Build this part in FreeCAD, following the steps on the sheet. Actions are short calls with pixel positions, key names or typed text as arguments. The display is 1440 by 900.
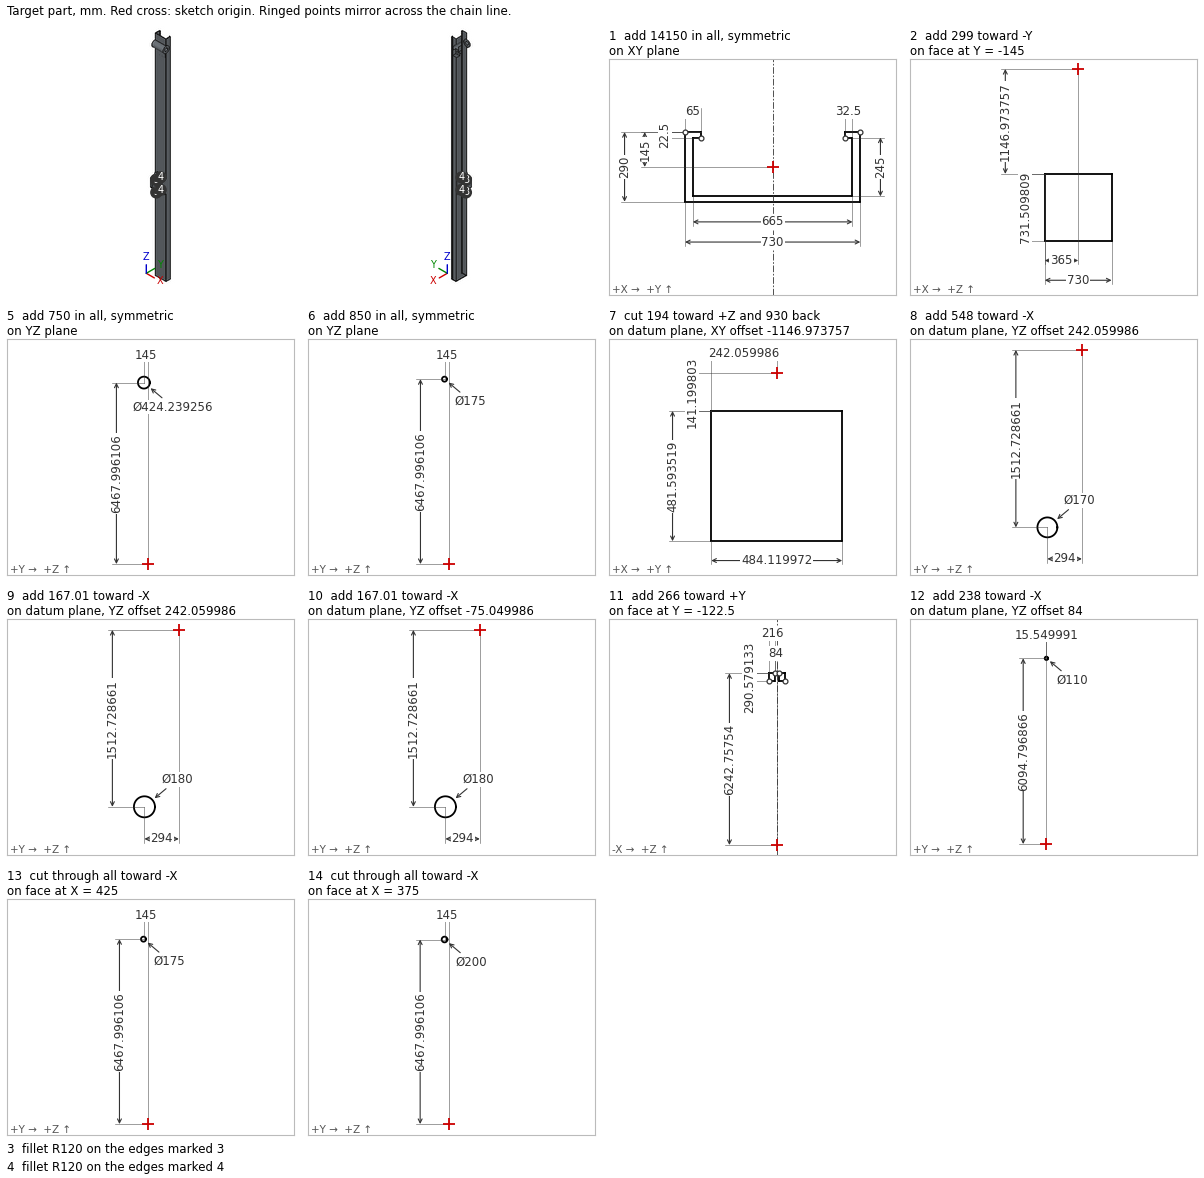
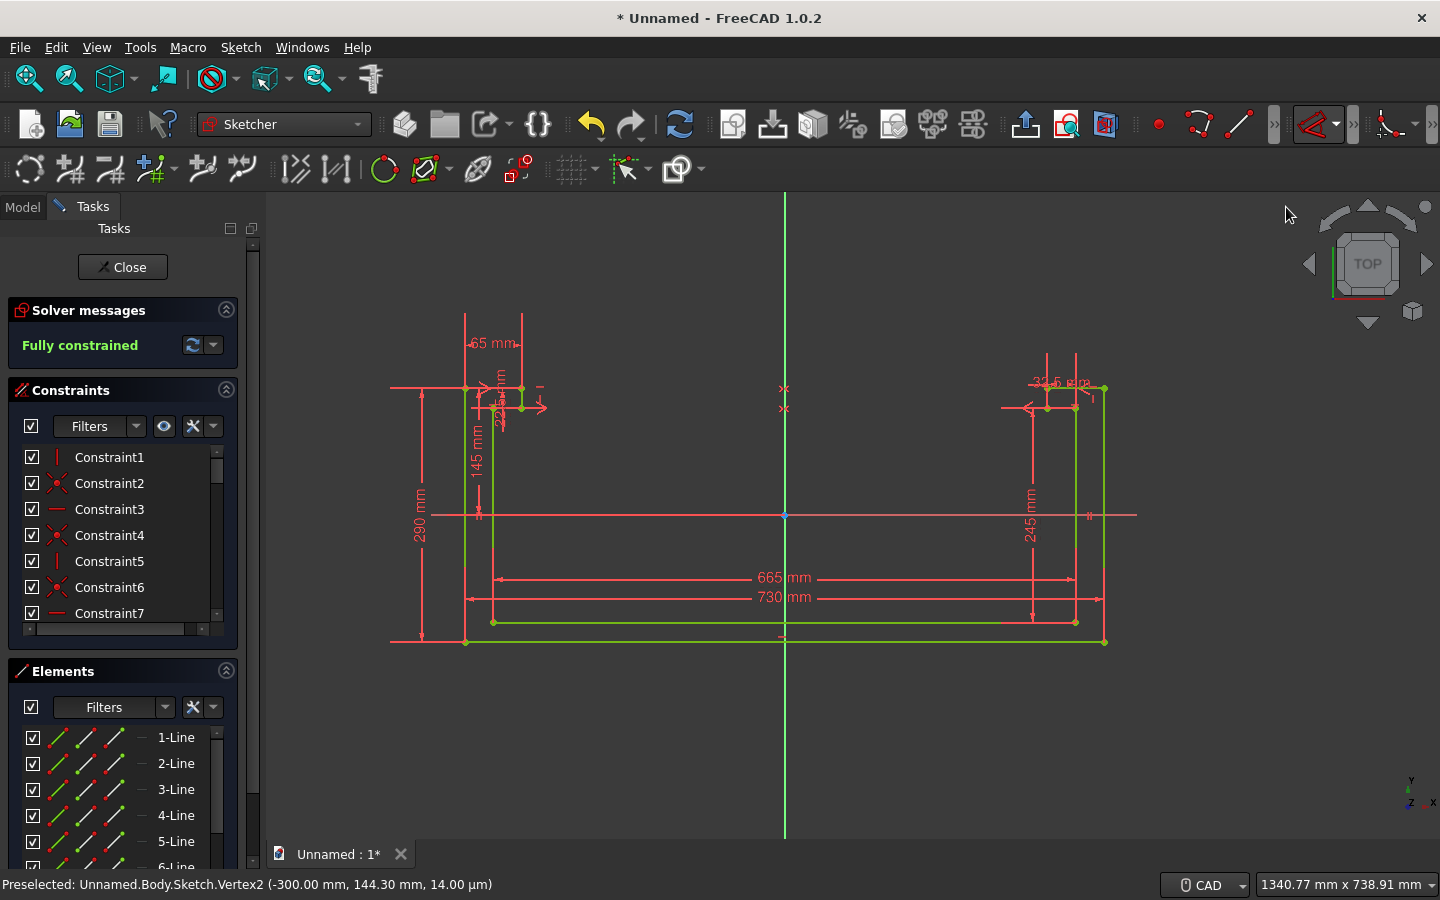
click(123, 267)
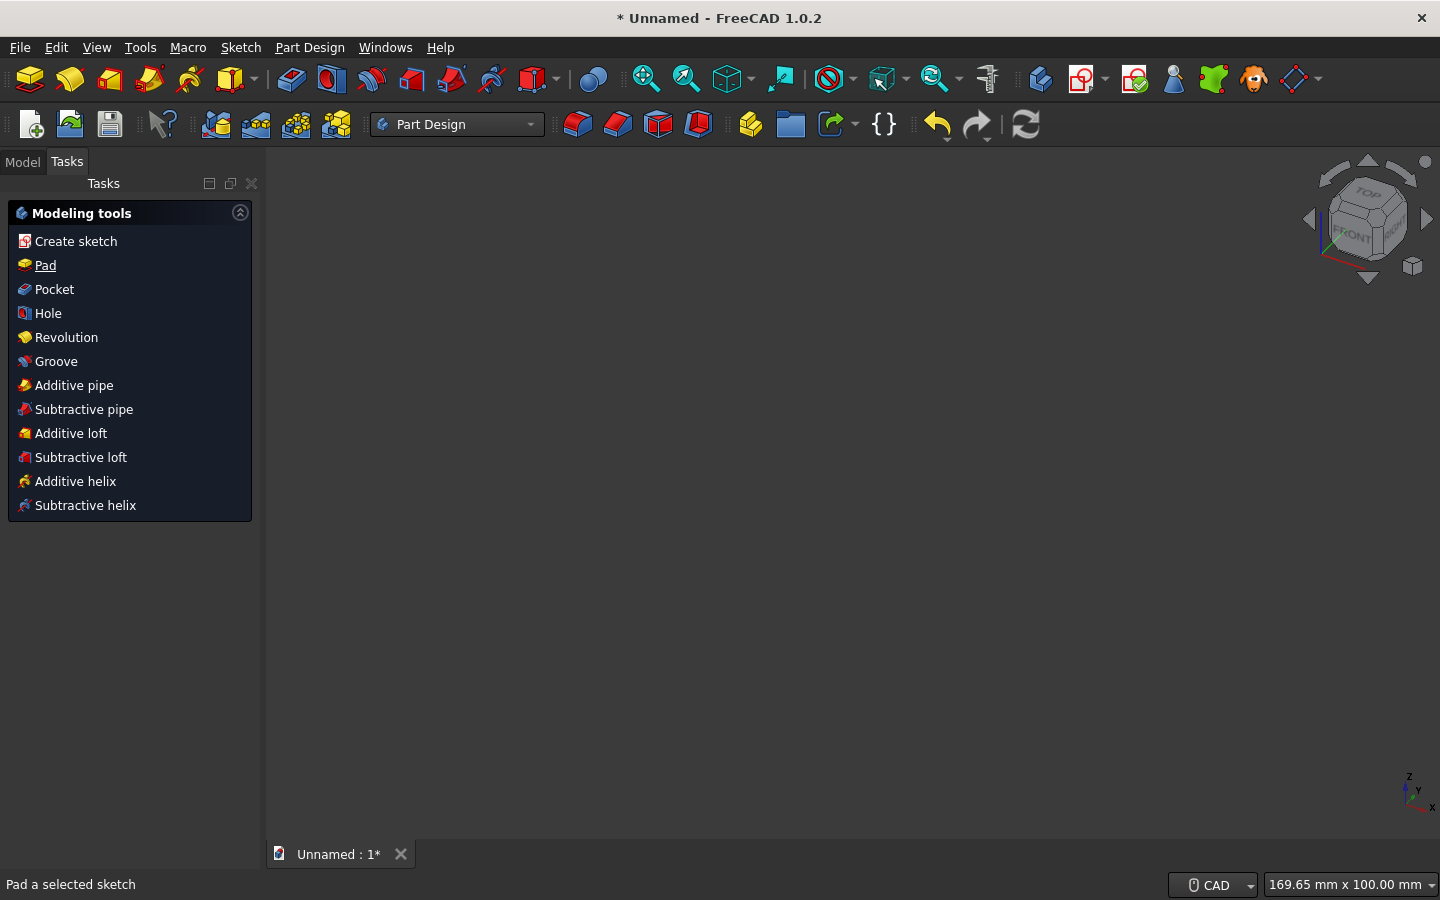
click(30, 80)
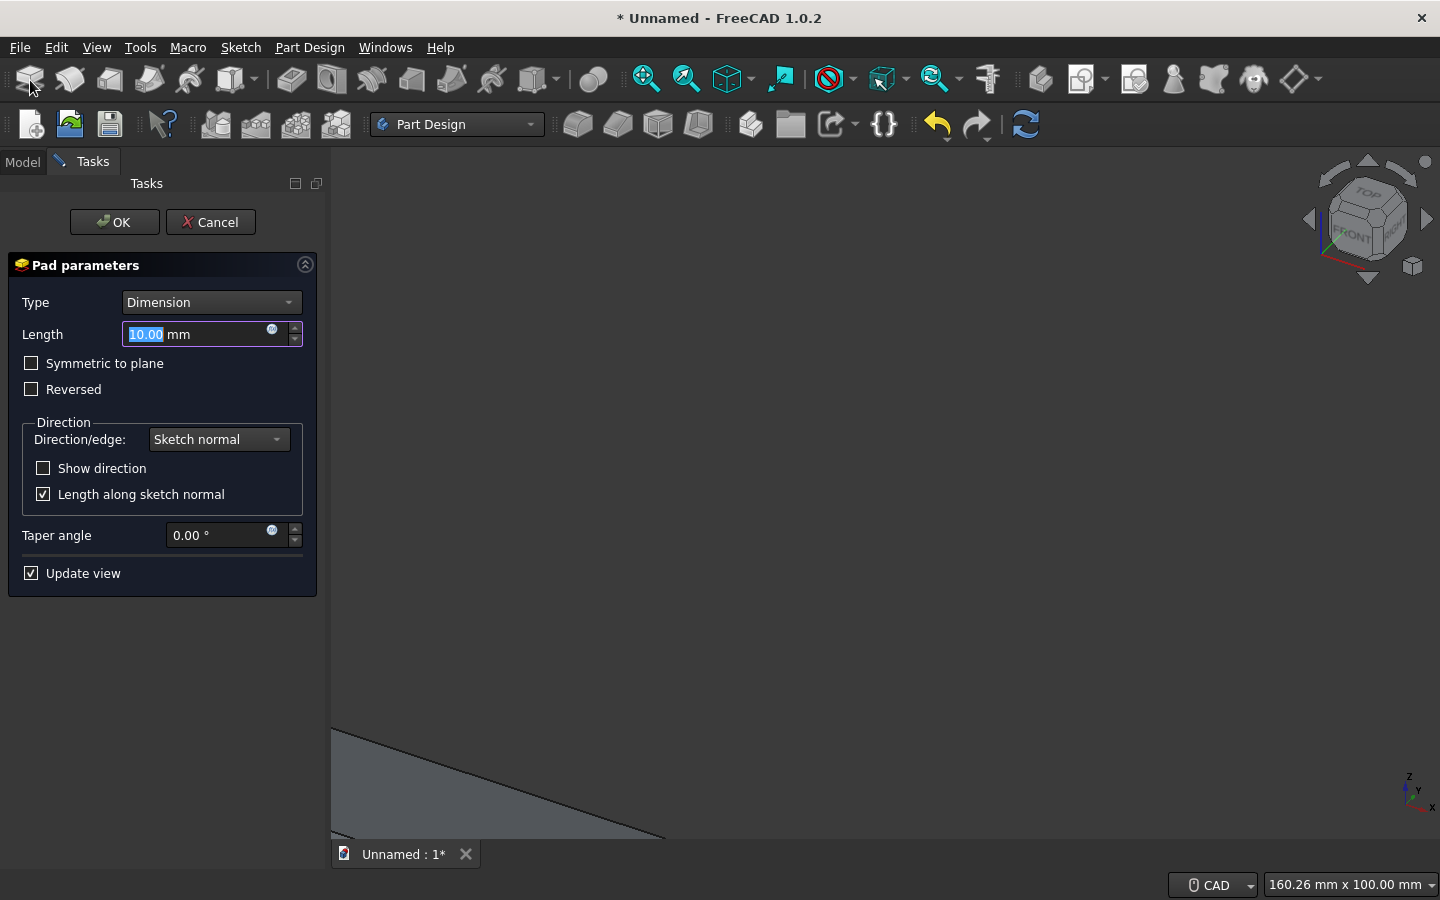
text(14150)
key(Tab)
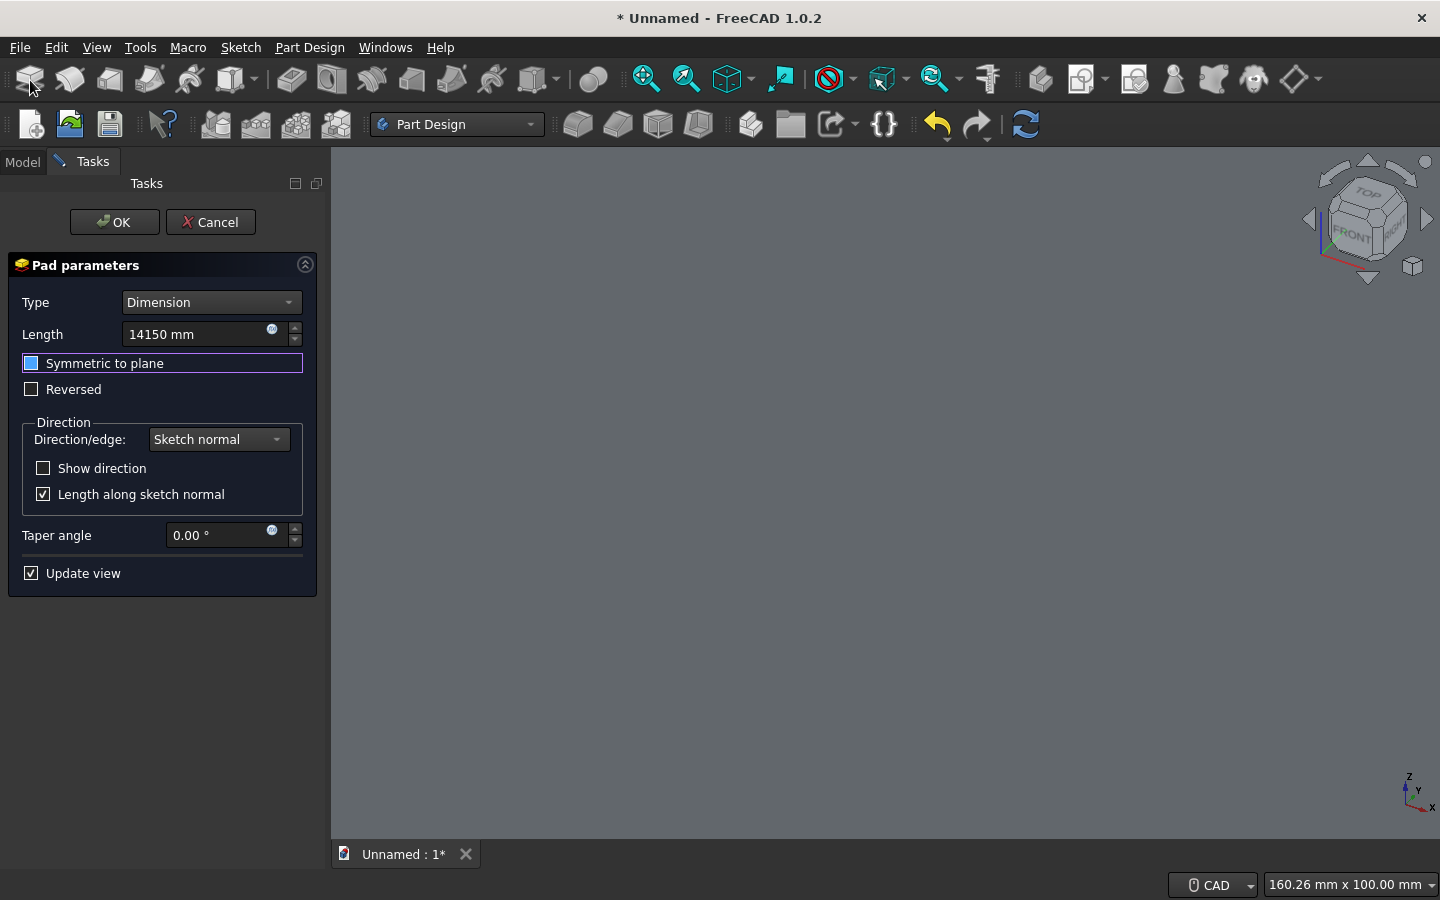
click(30, 363)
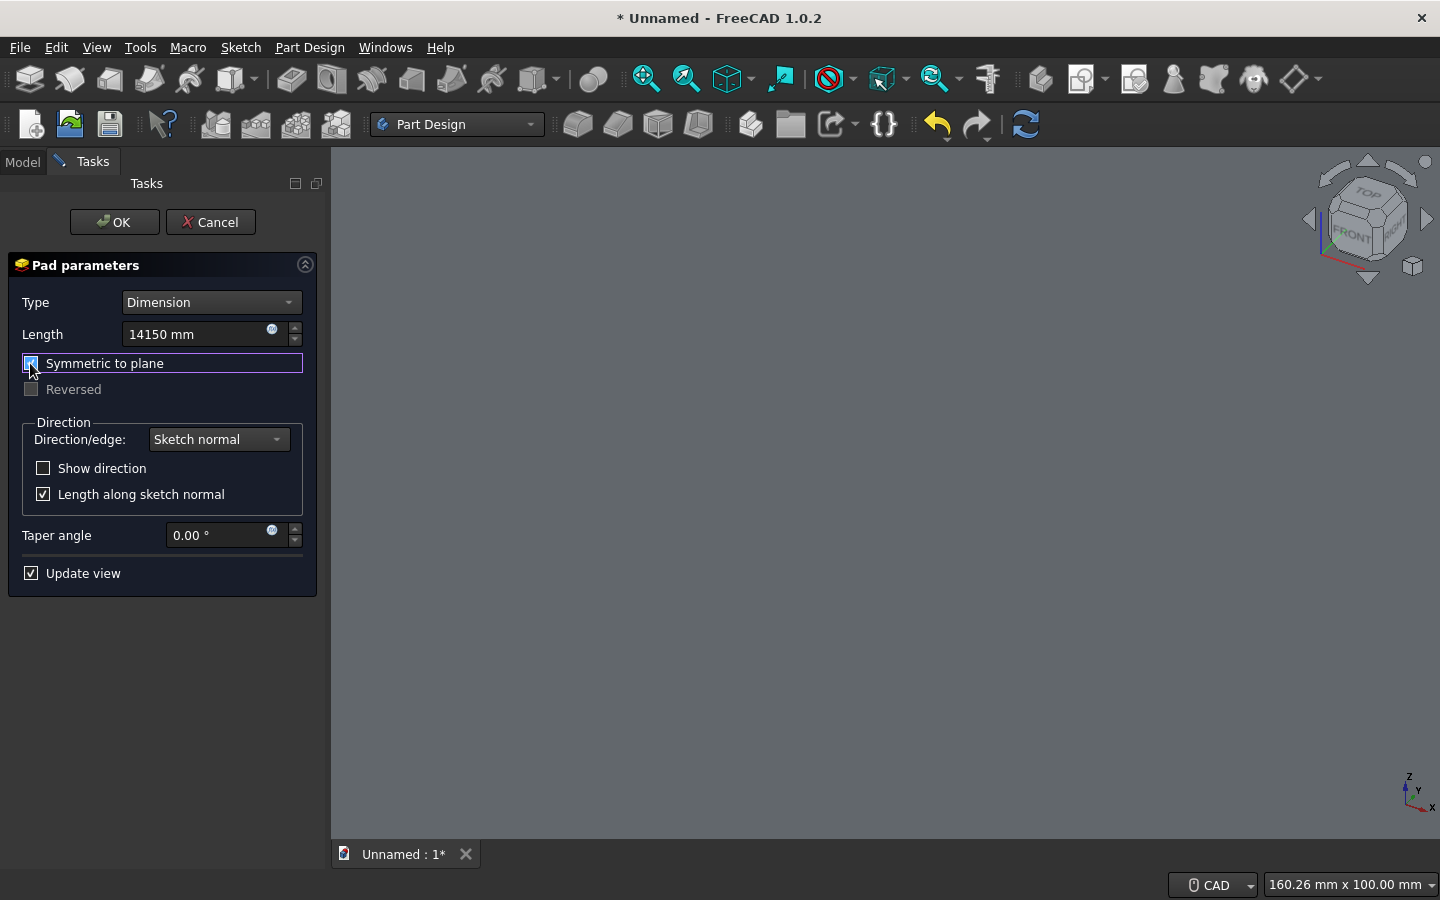
click(115, 222)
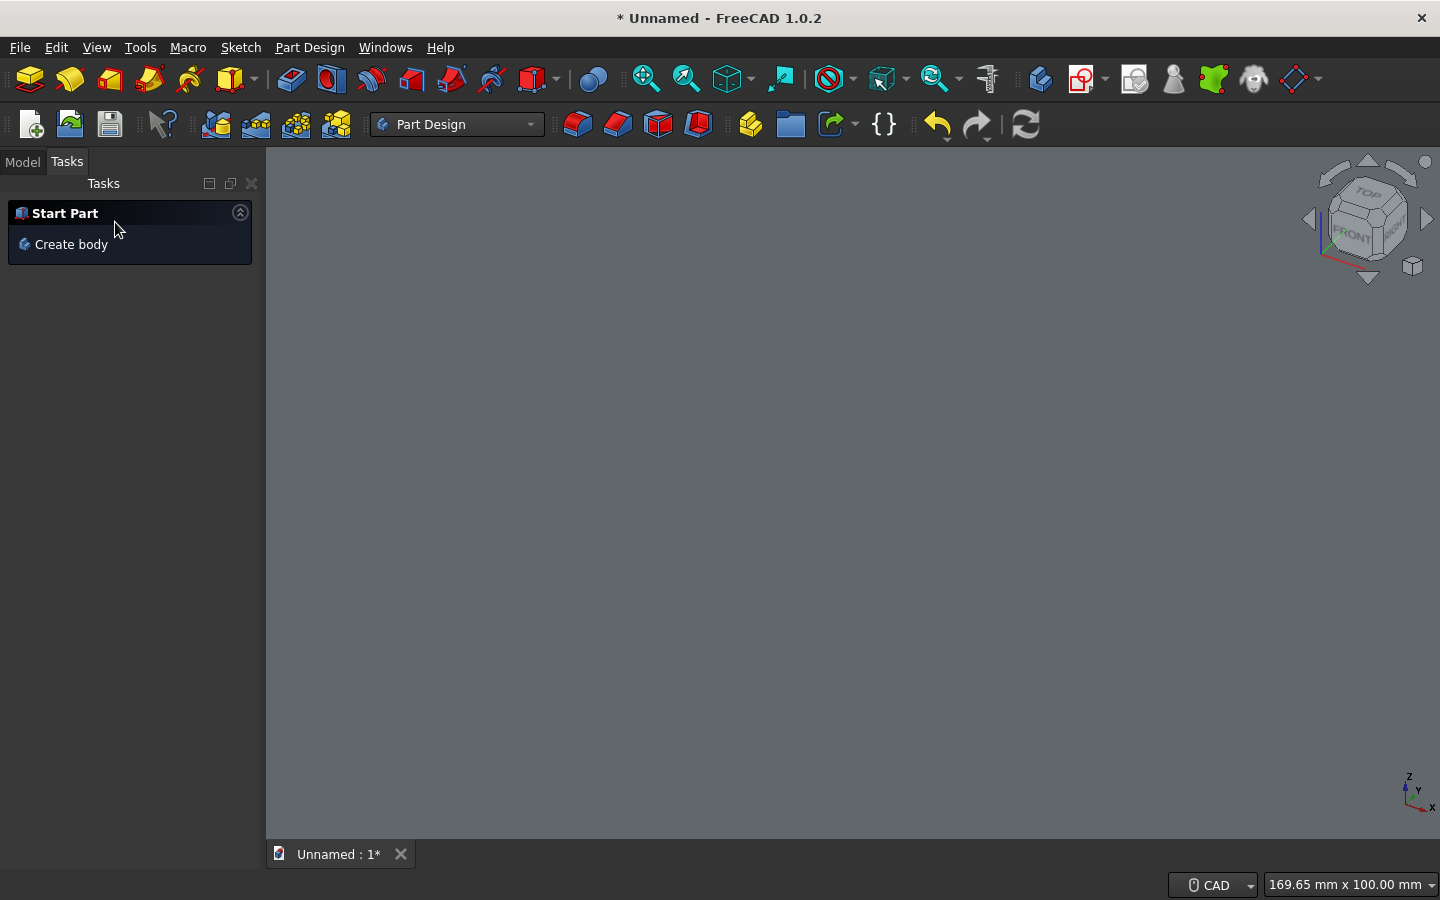
key(v)
key(f)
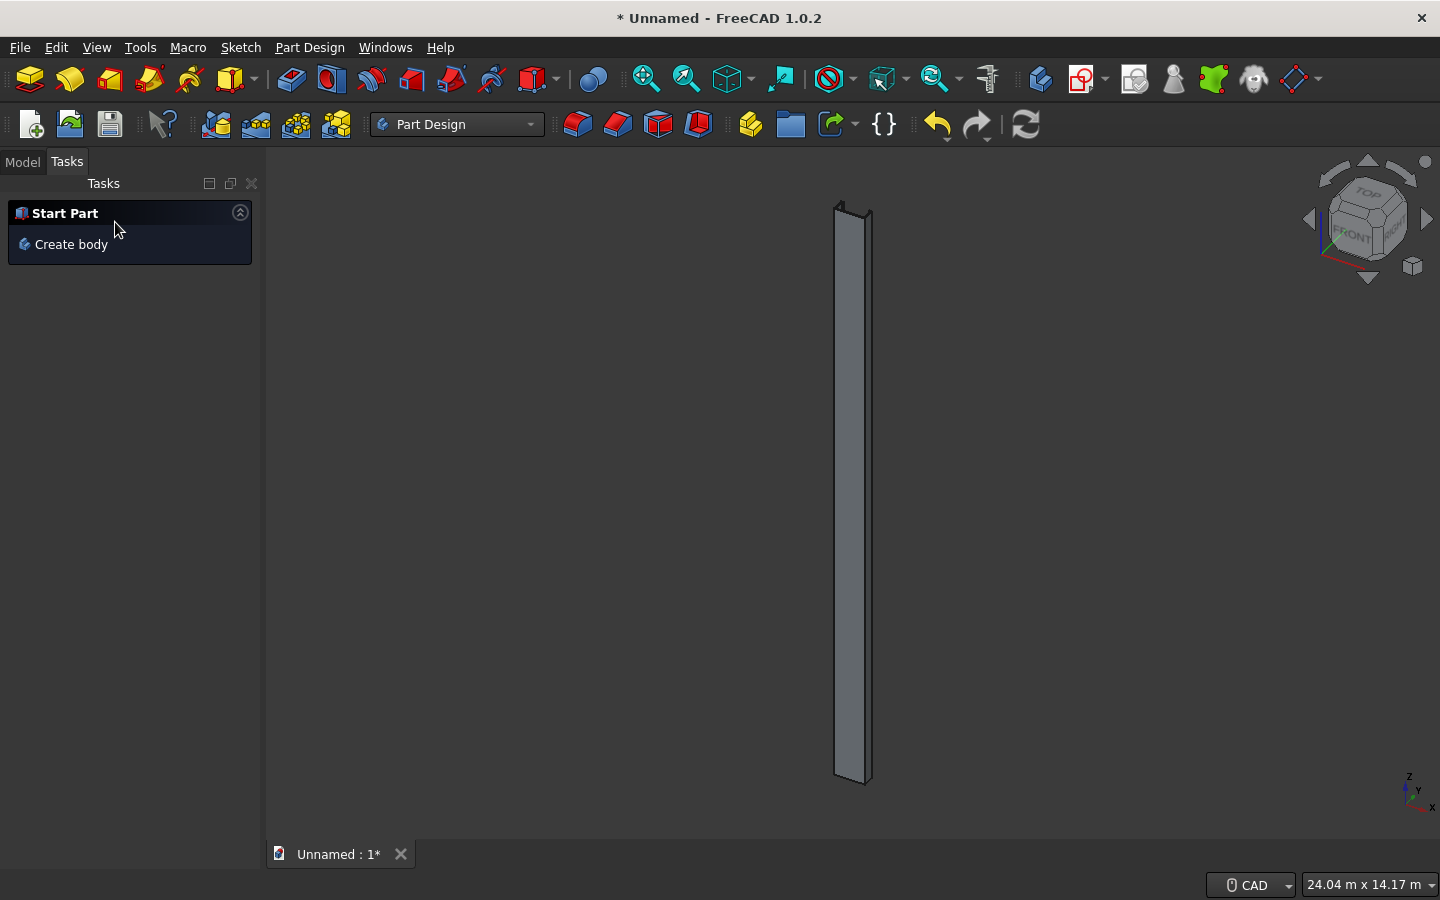
click(849, 253)